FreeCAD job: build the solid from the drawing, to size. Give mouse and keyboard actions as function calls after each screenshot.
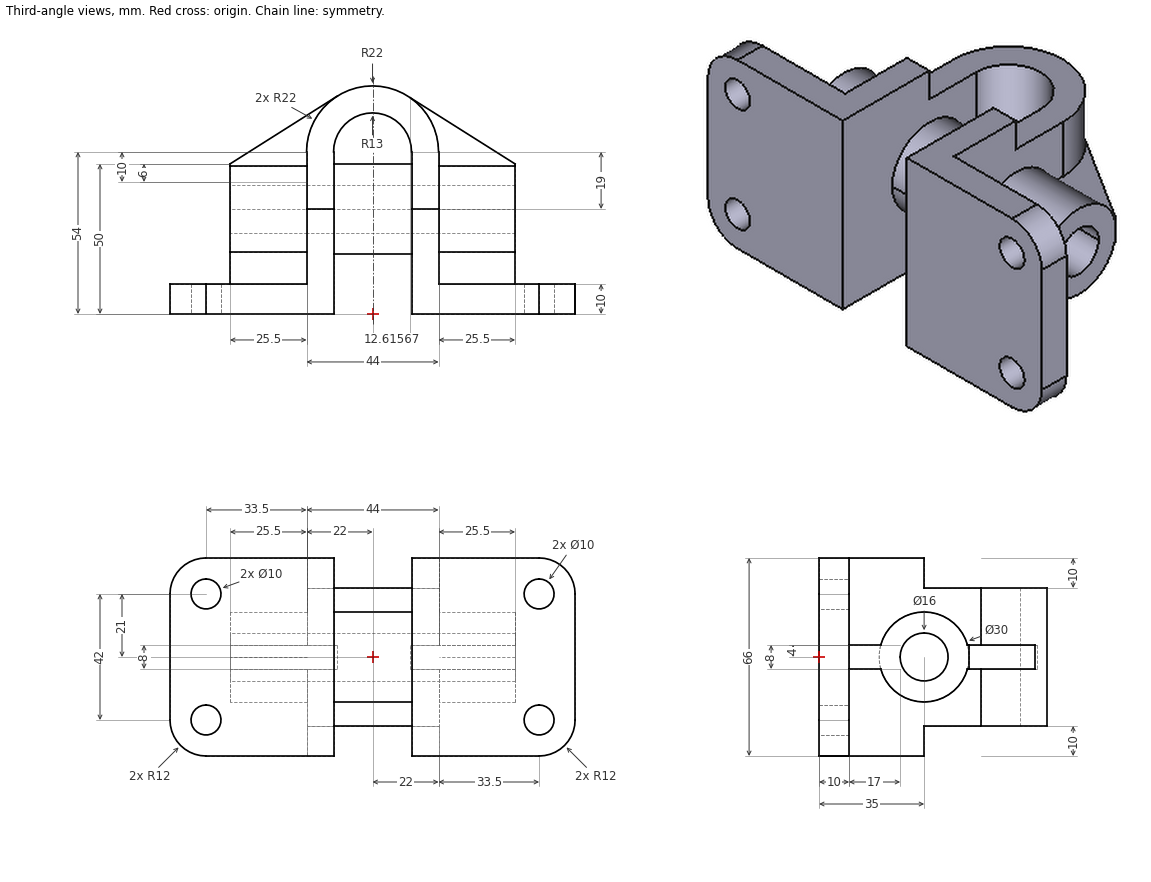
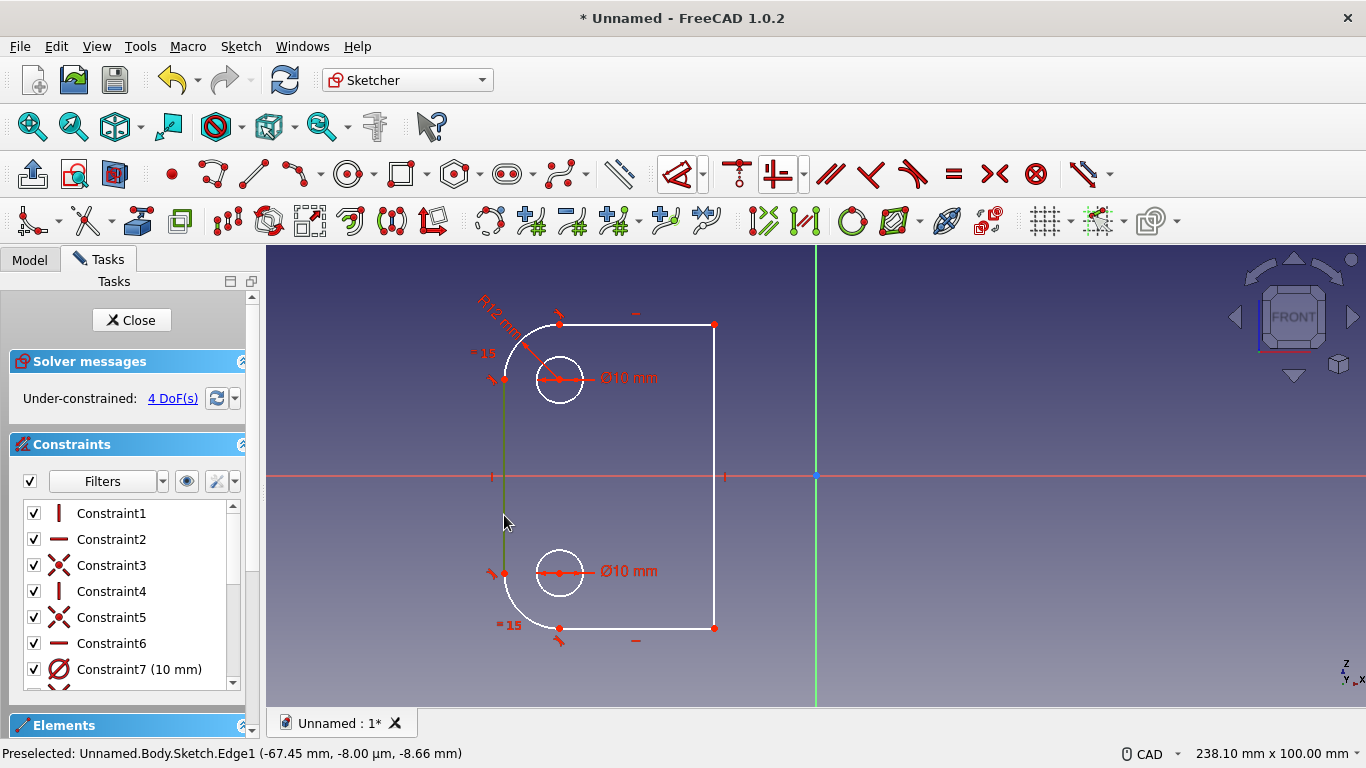
click(702, 174)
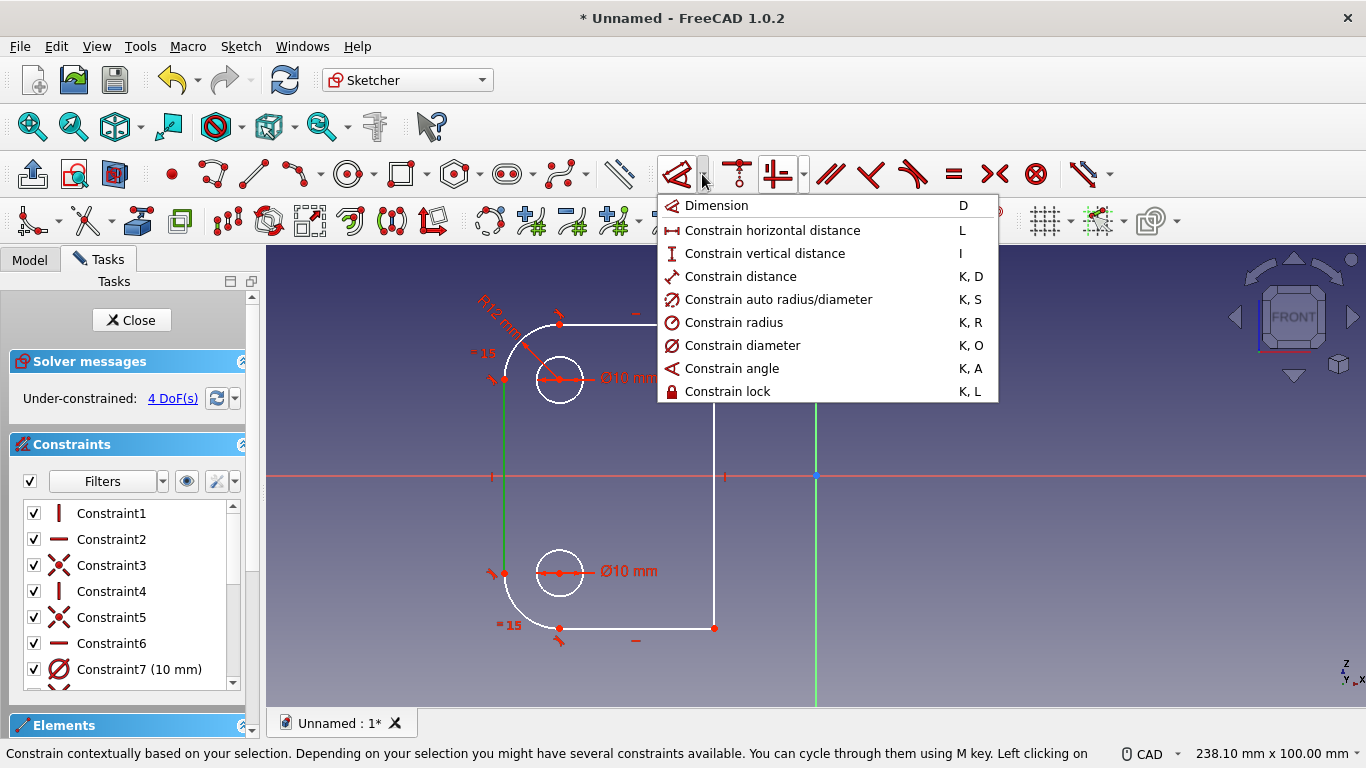
click(828, 254)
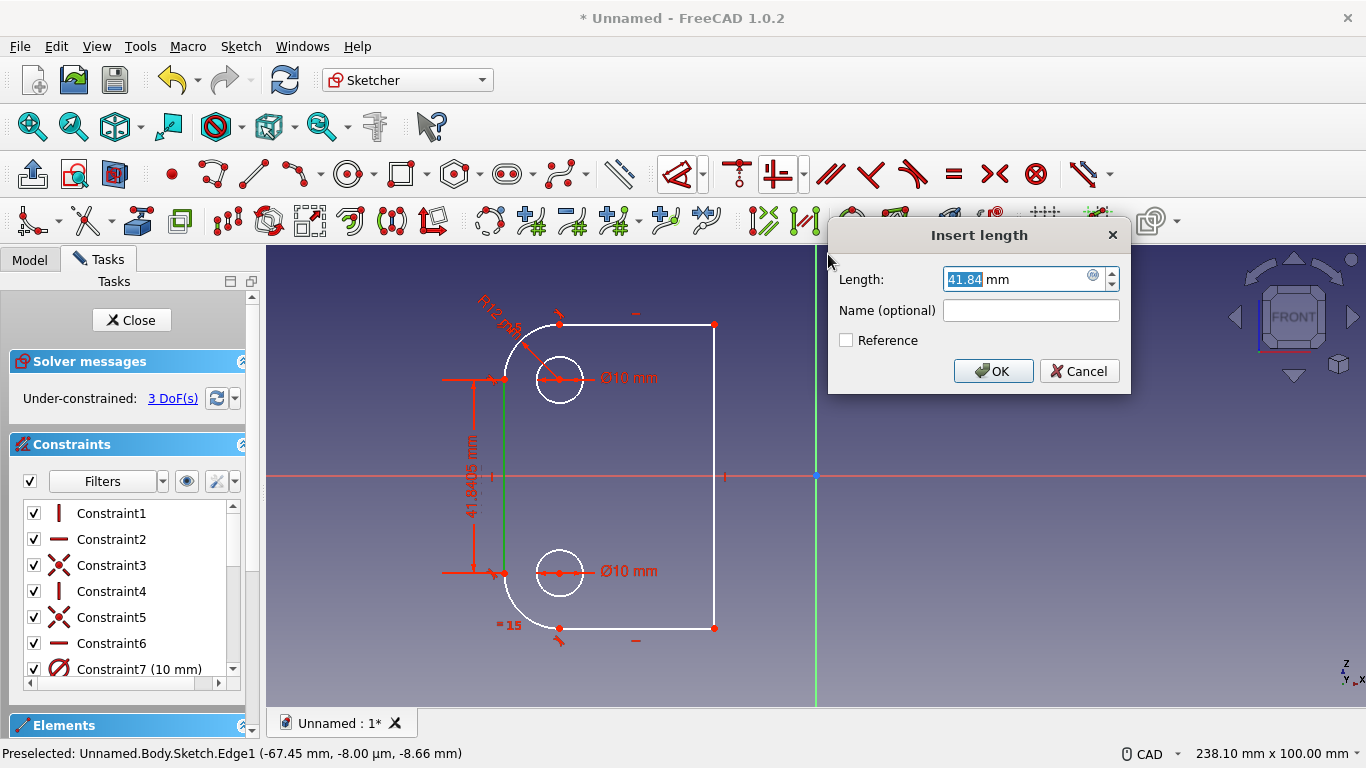
text(42)
key(Return)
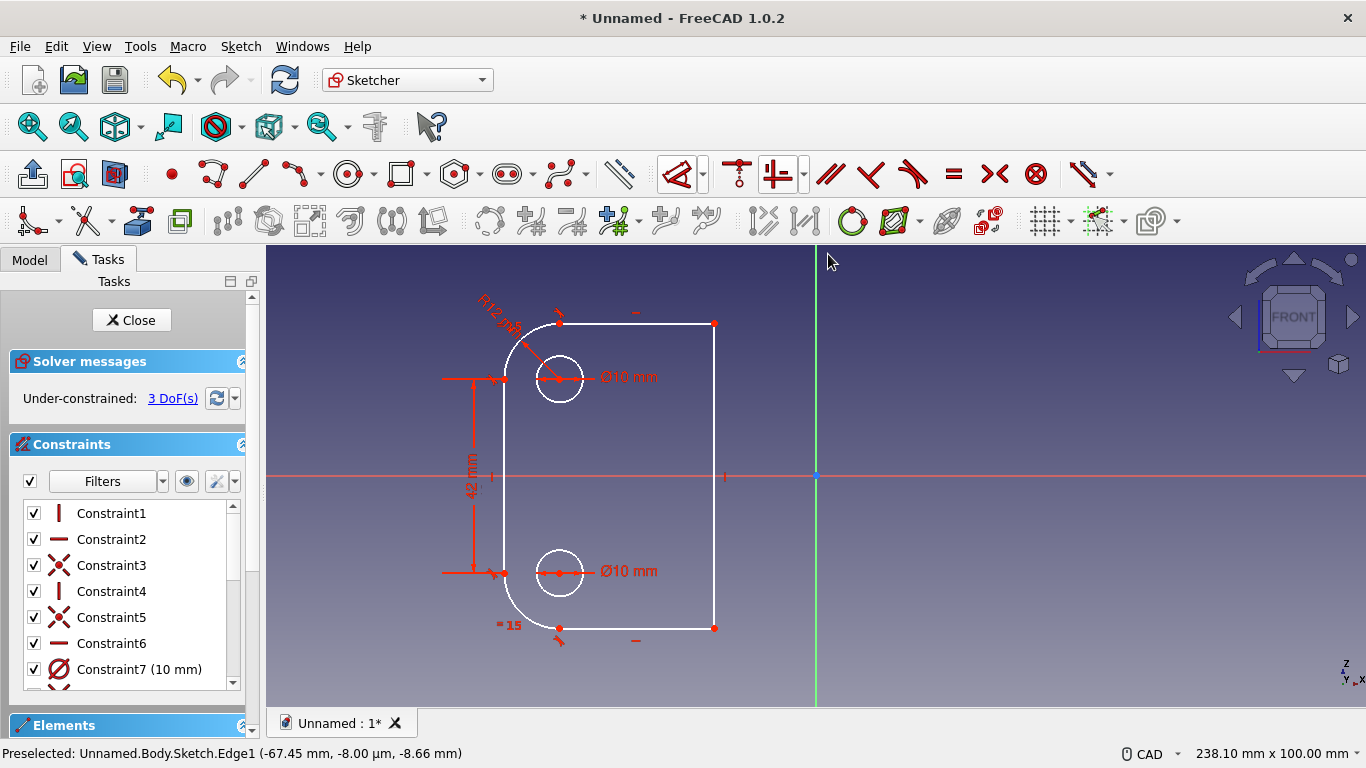
click(560, 379)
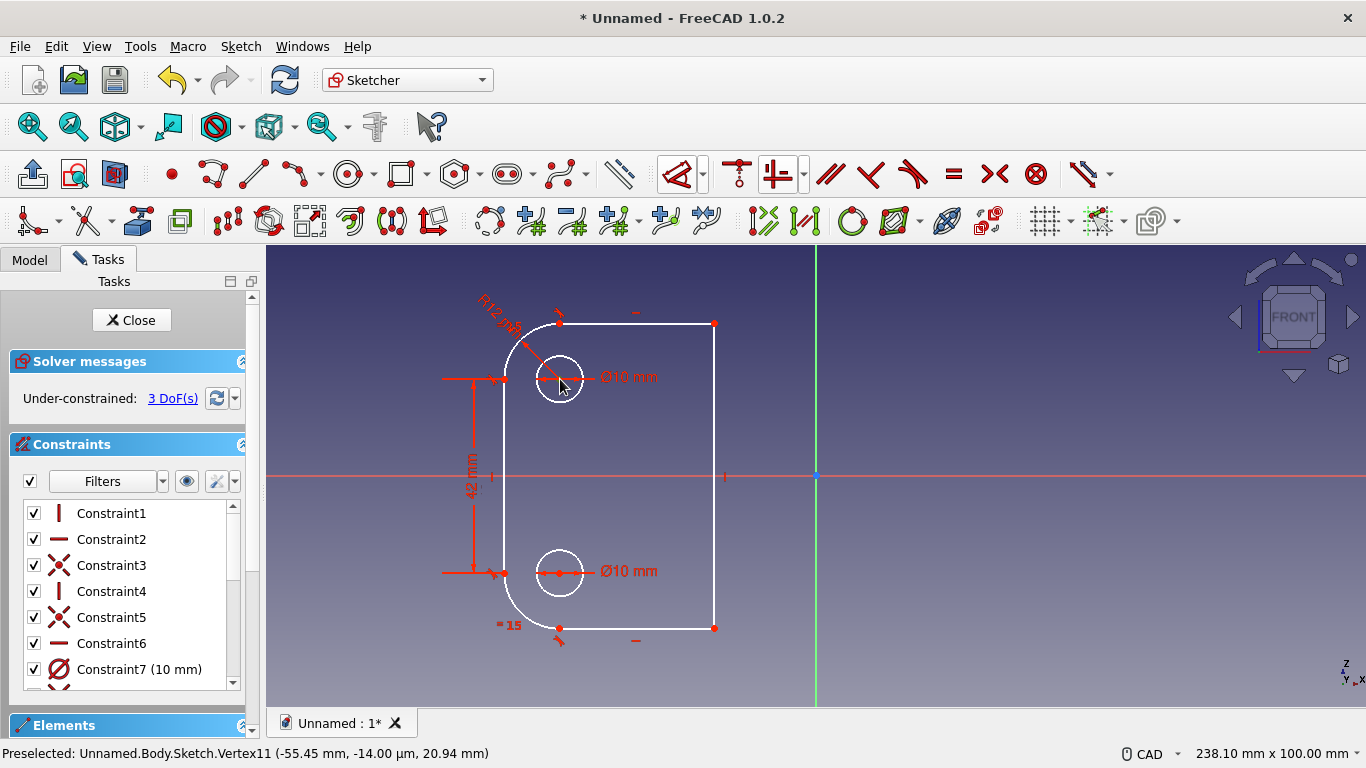
key(i)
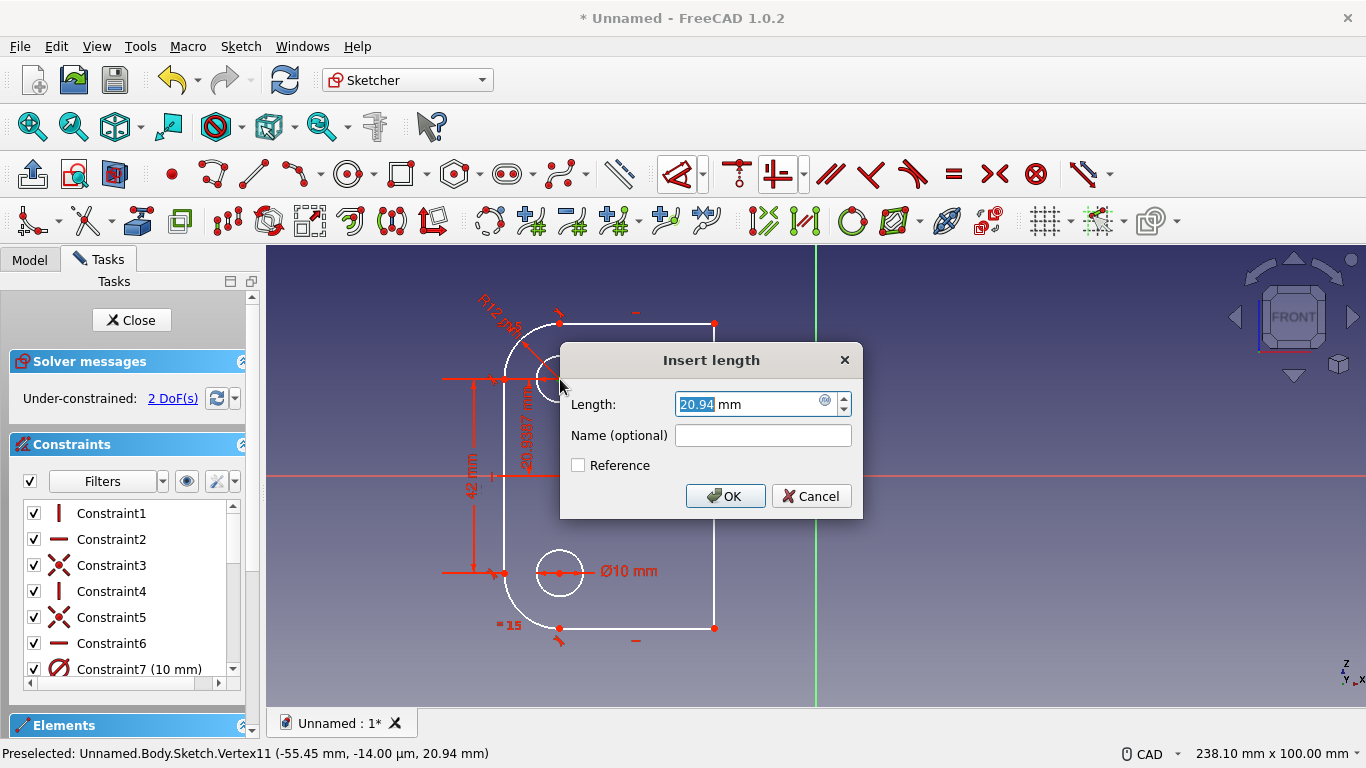
text(21)
key(Return)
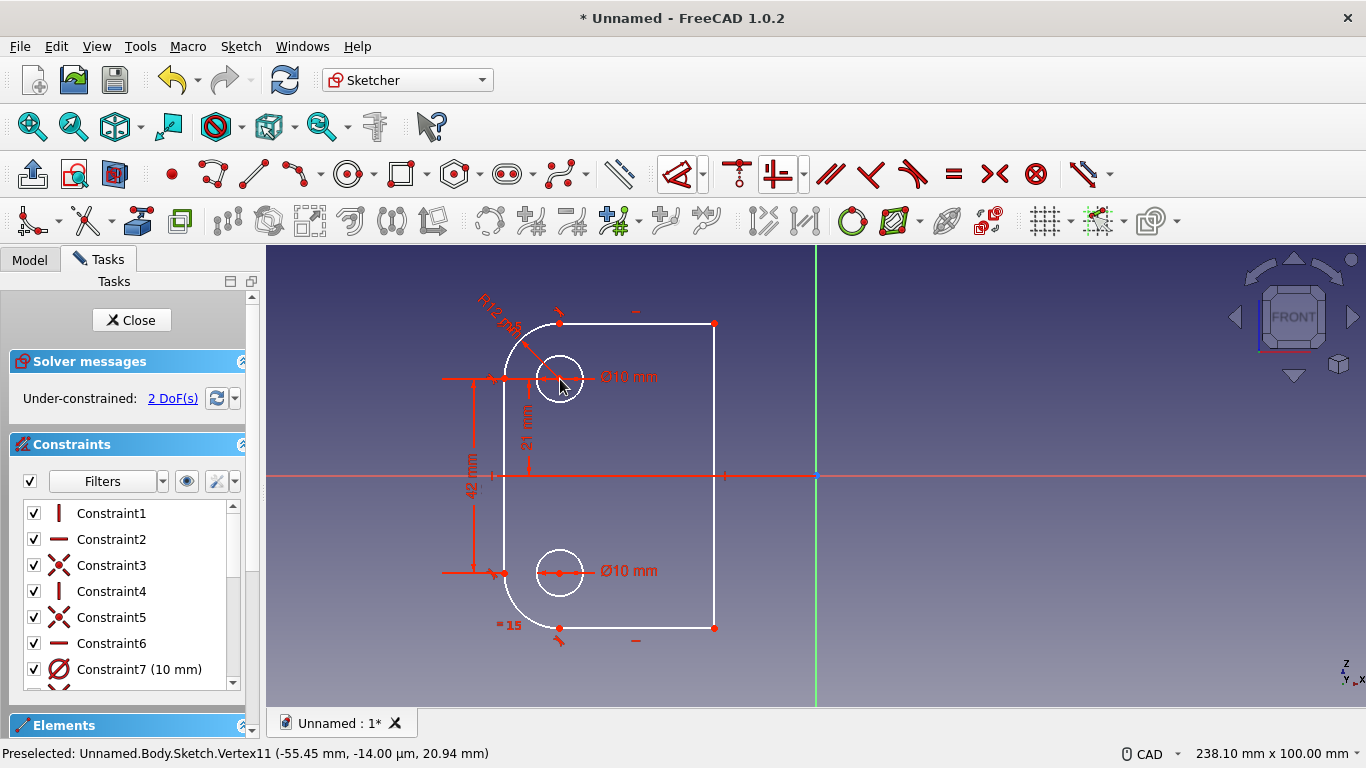
click(714, 324)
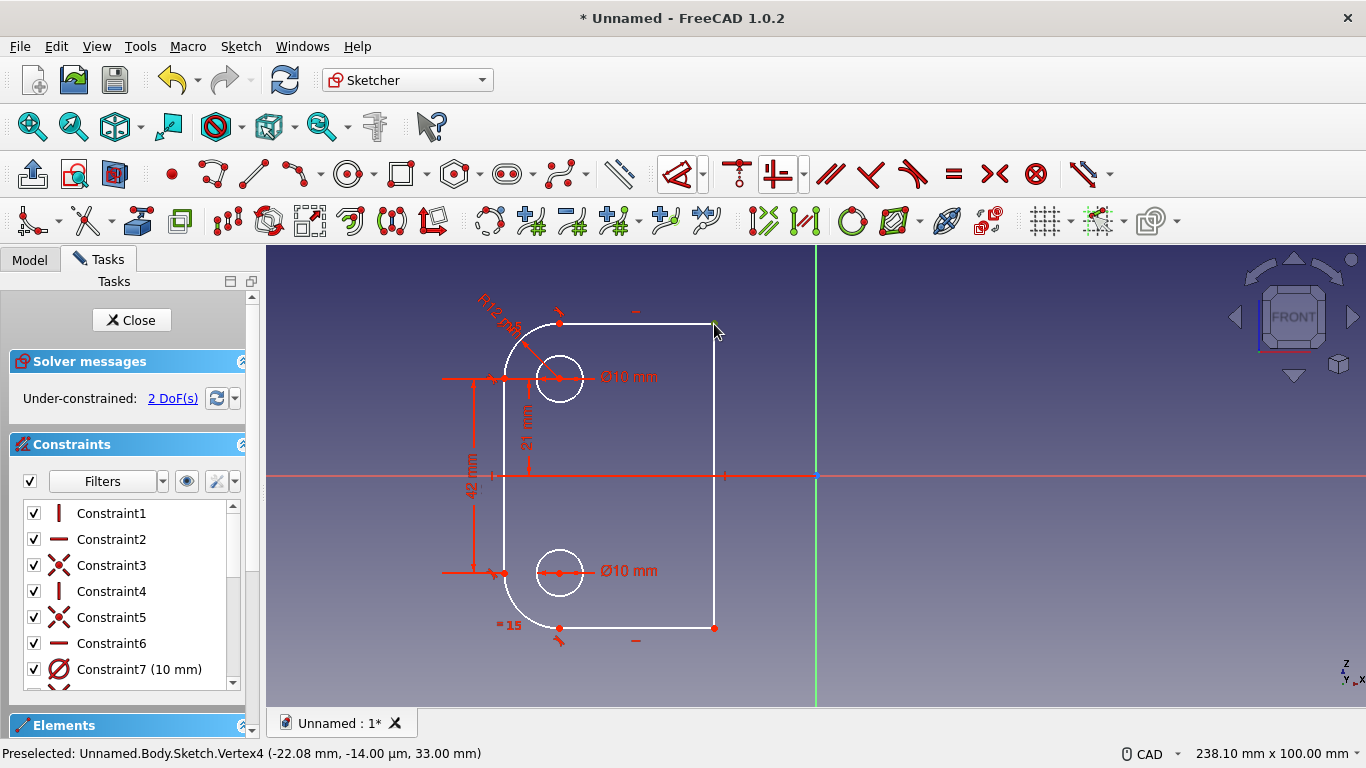
click(702, 174)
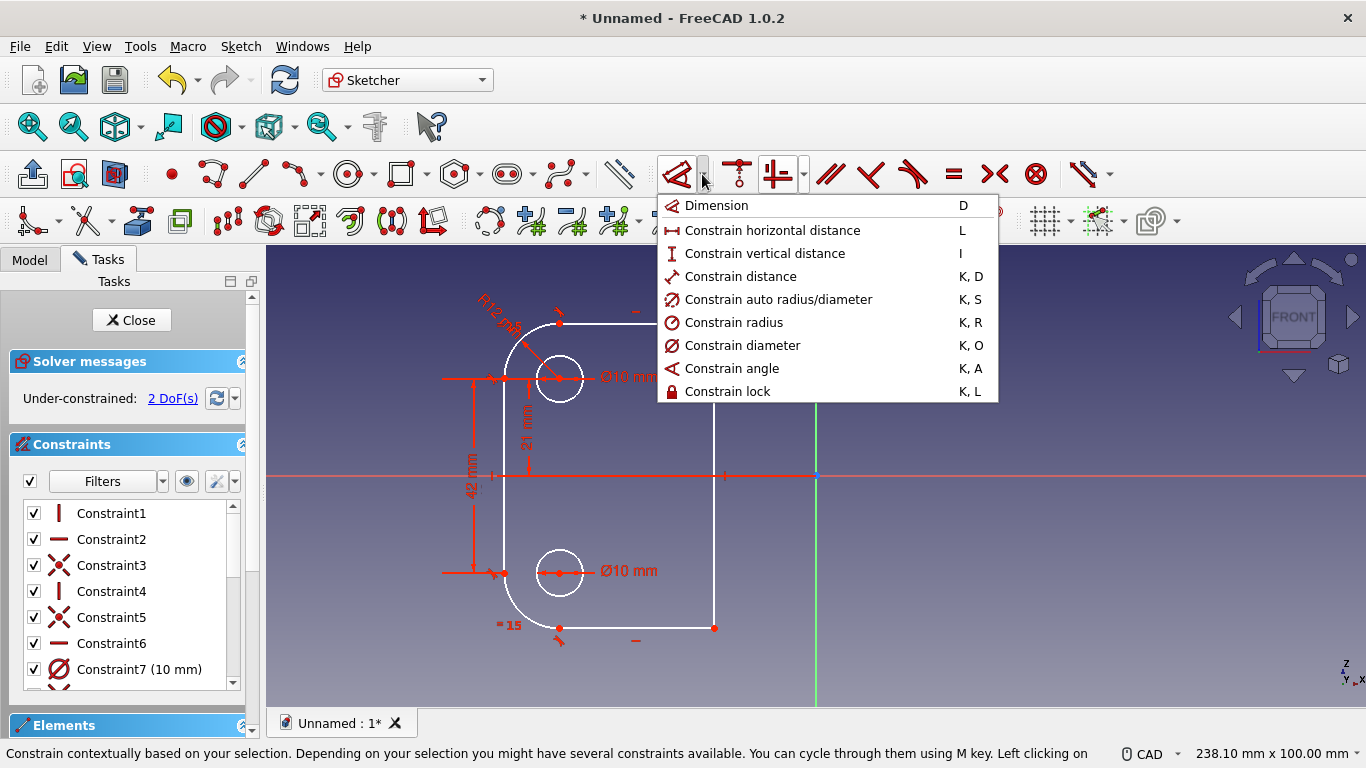
click(828, 230)